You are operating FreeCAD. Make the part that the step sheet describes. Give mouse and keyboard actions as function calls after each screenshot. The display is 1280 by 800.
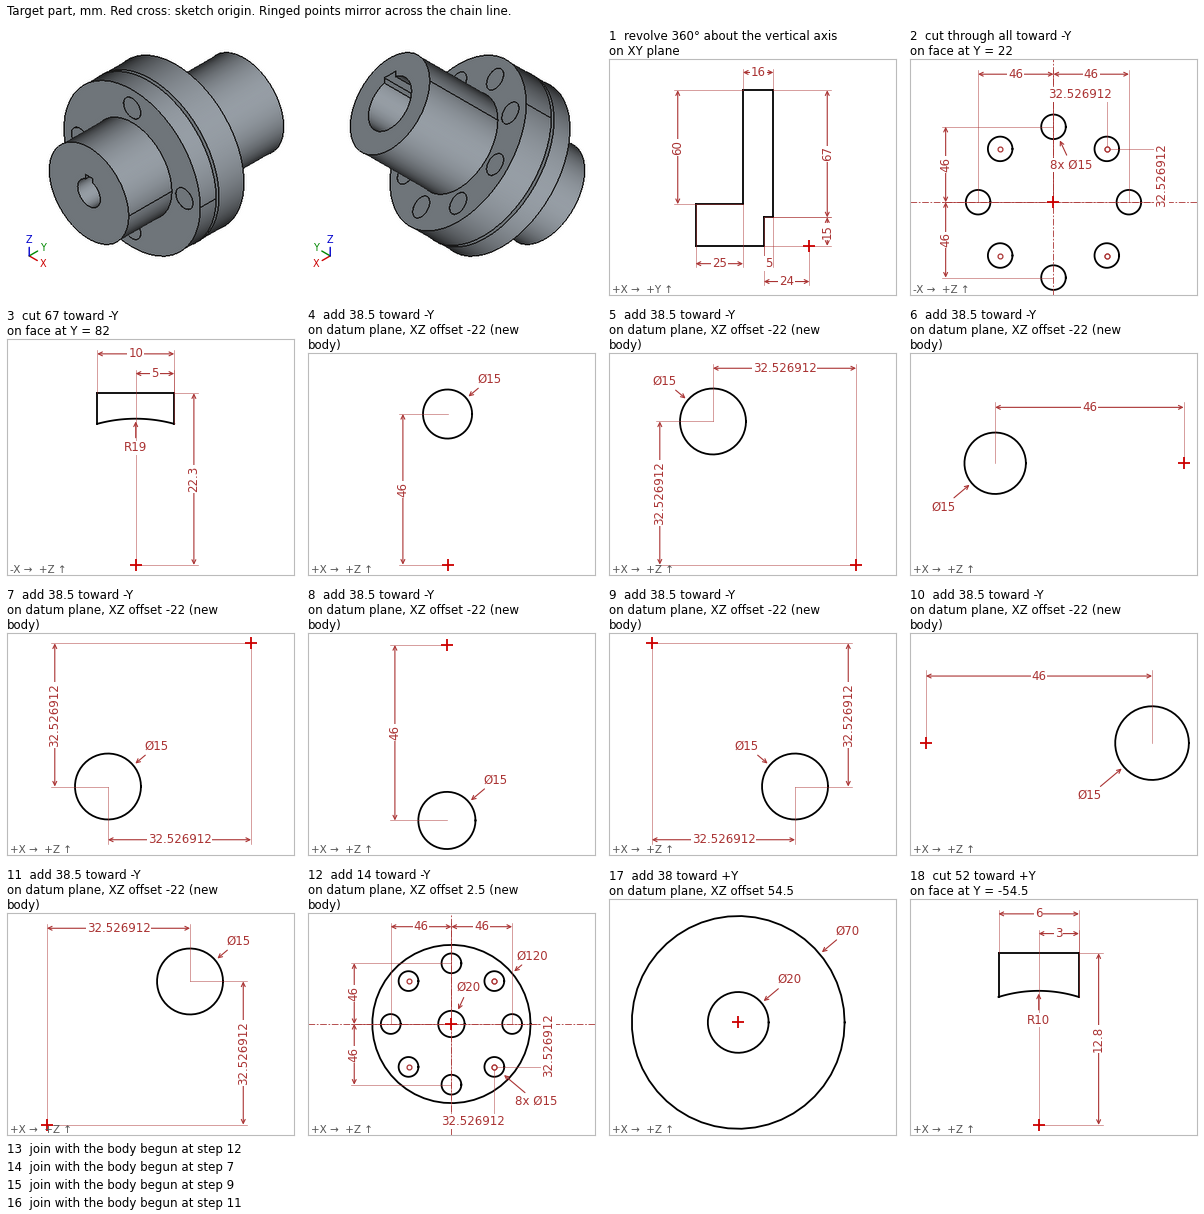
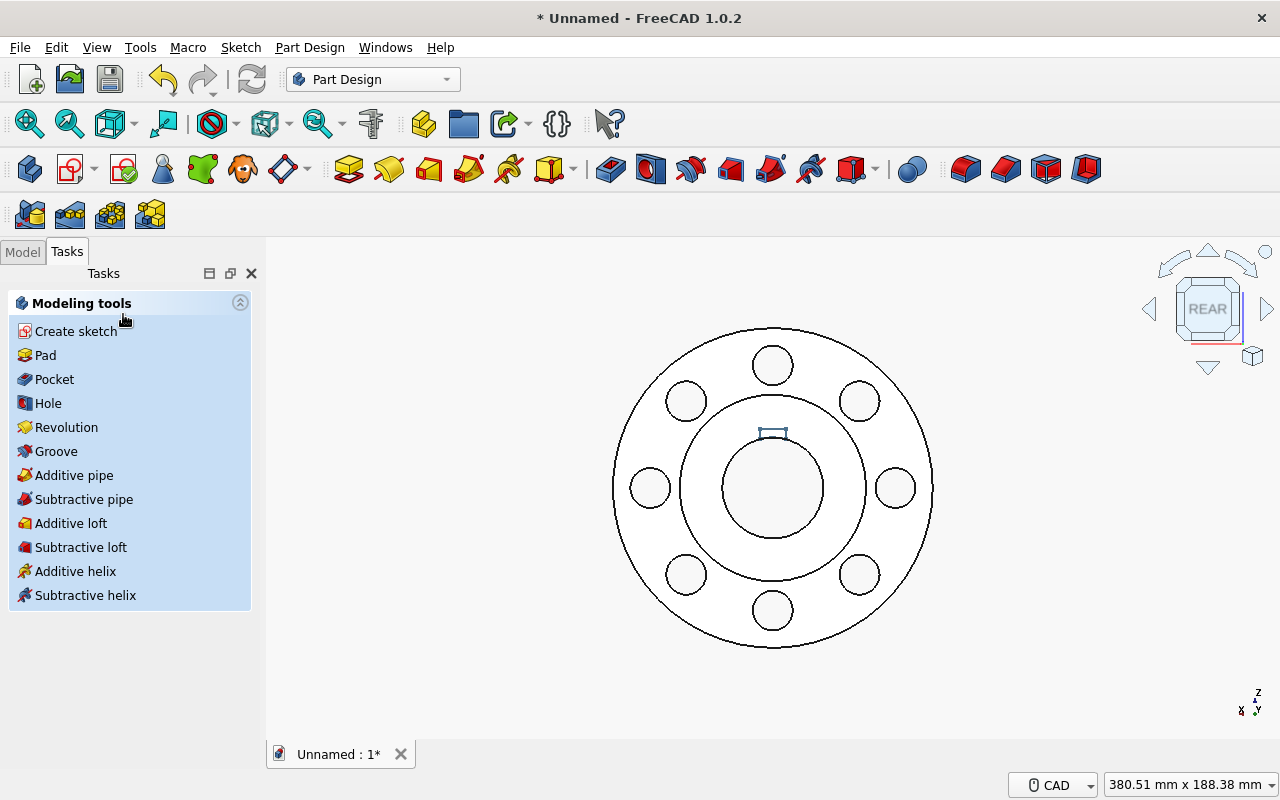
click(612, 170)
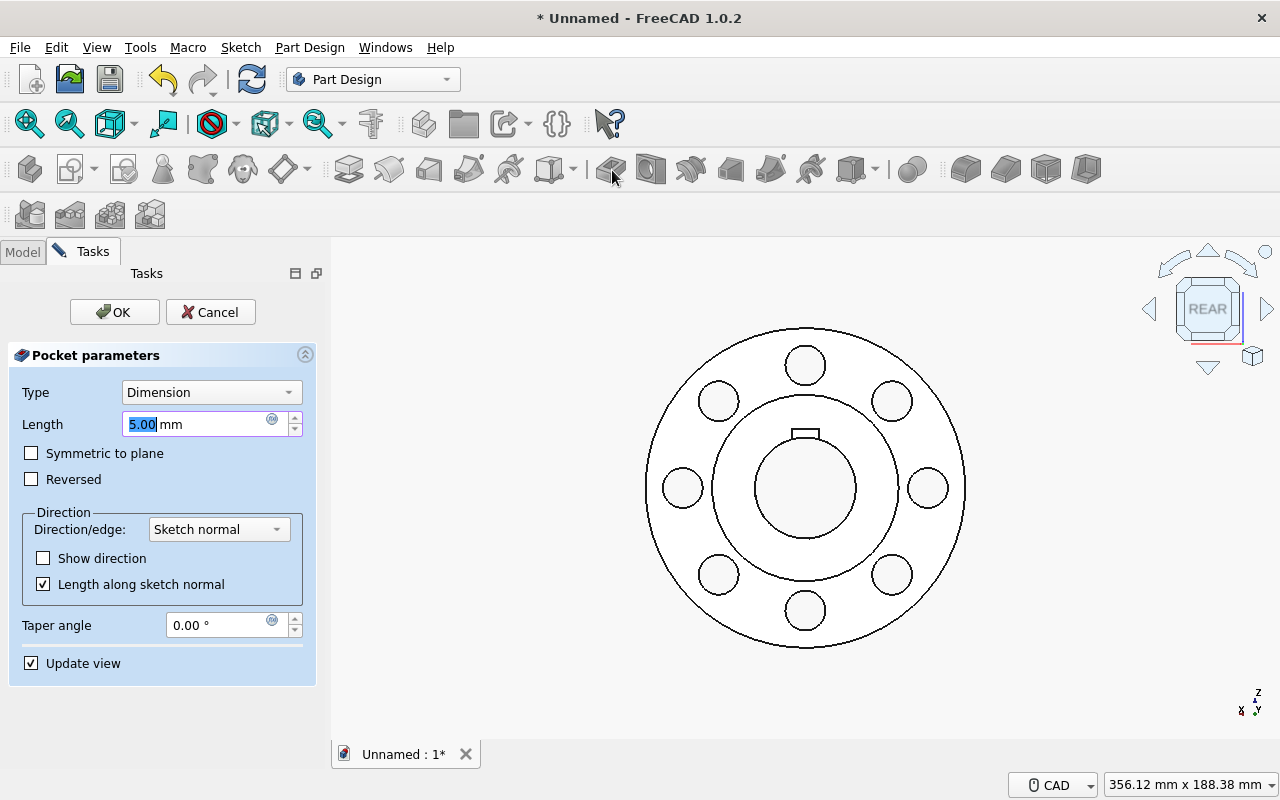
text(67)
key(Tab)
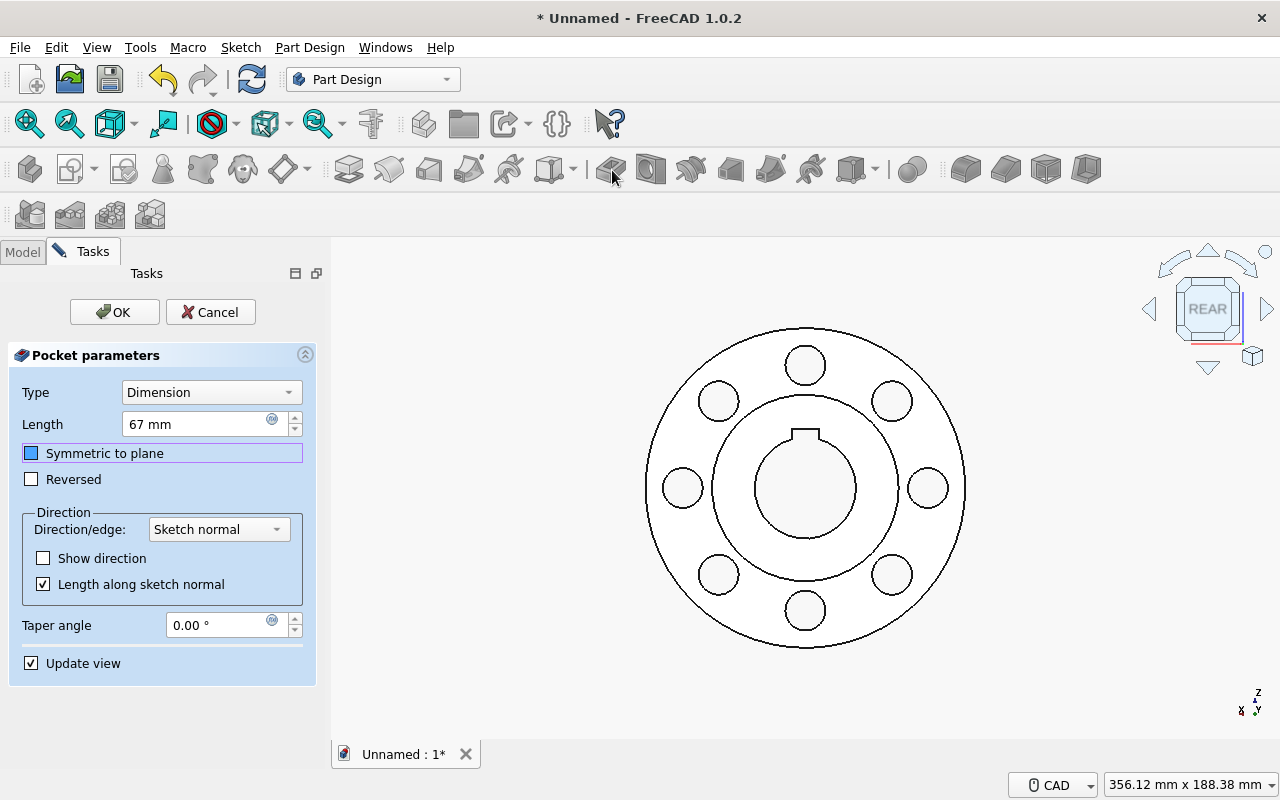
click(115, 312)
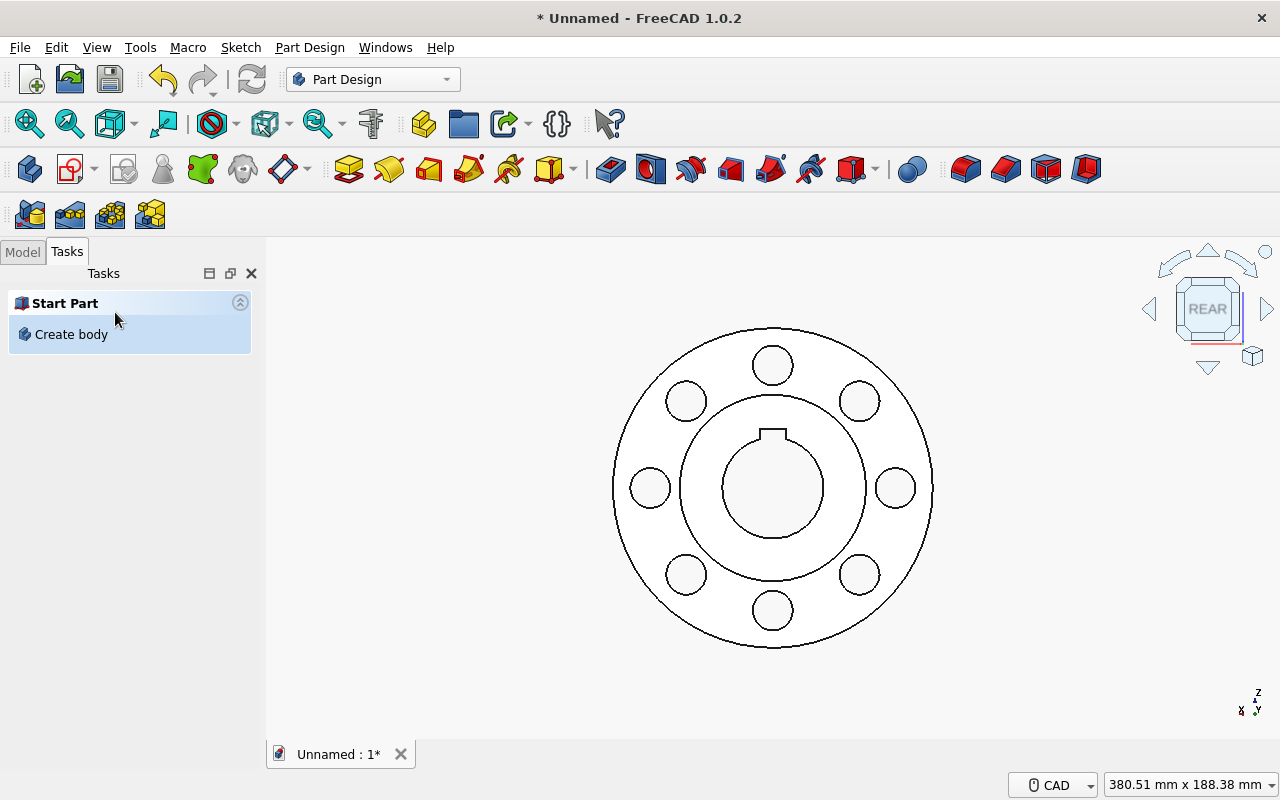
click(30, 170)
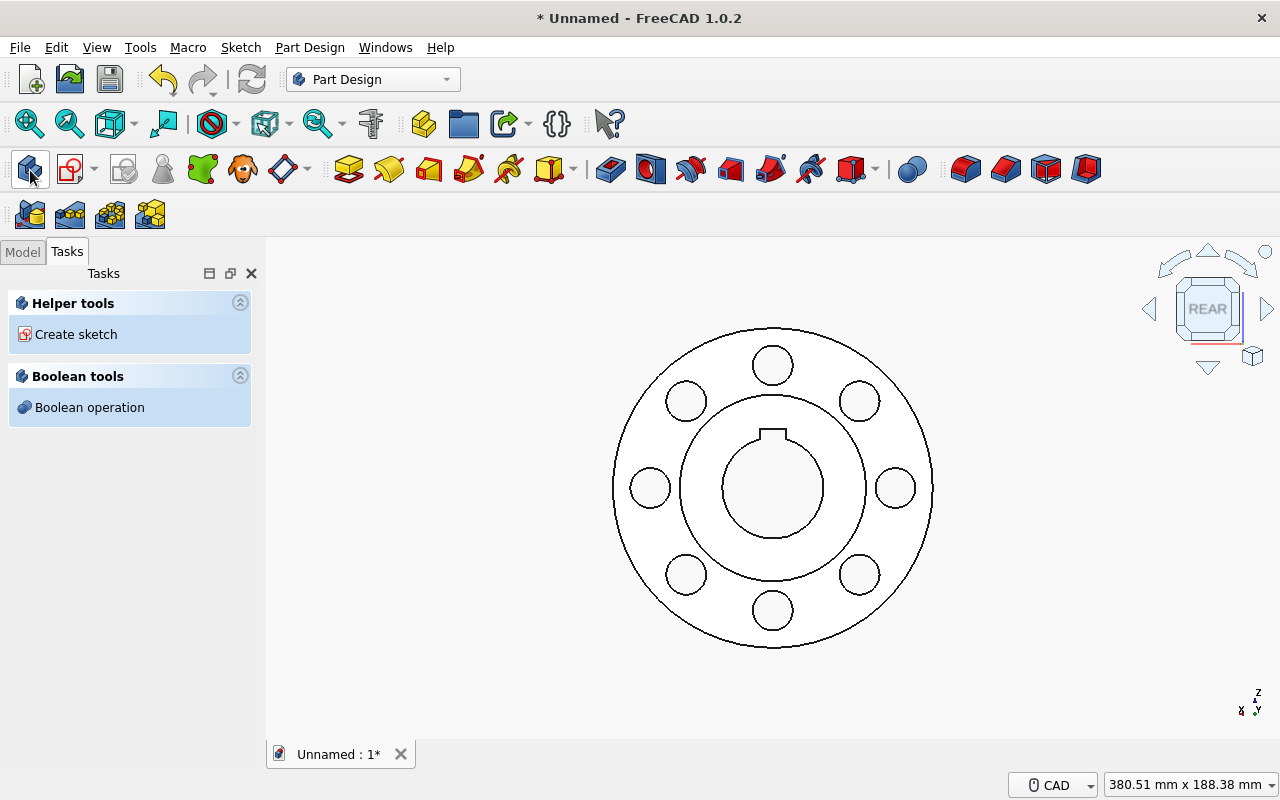
click(23, 251)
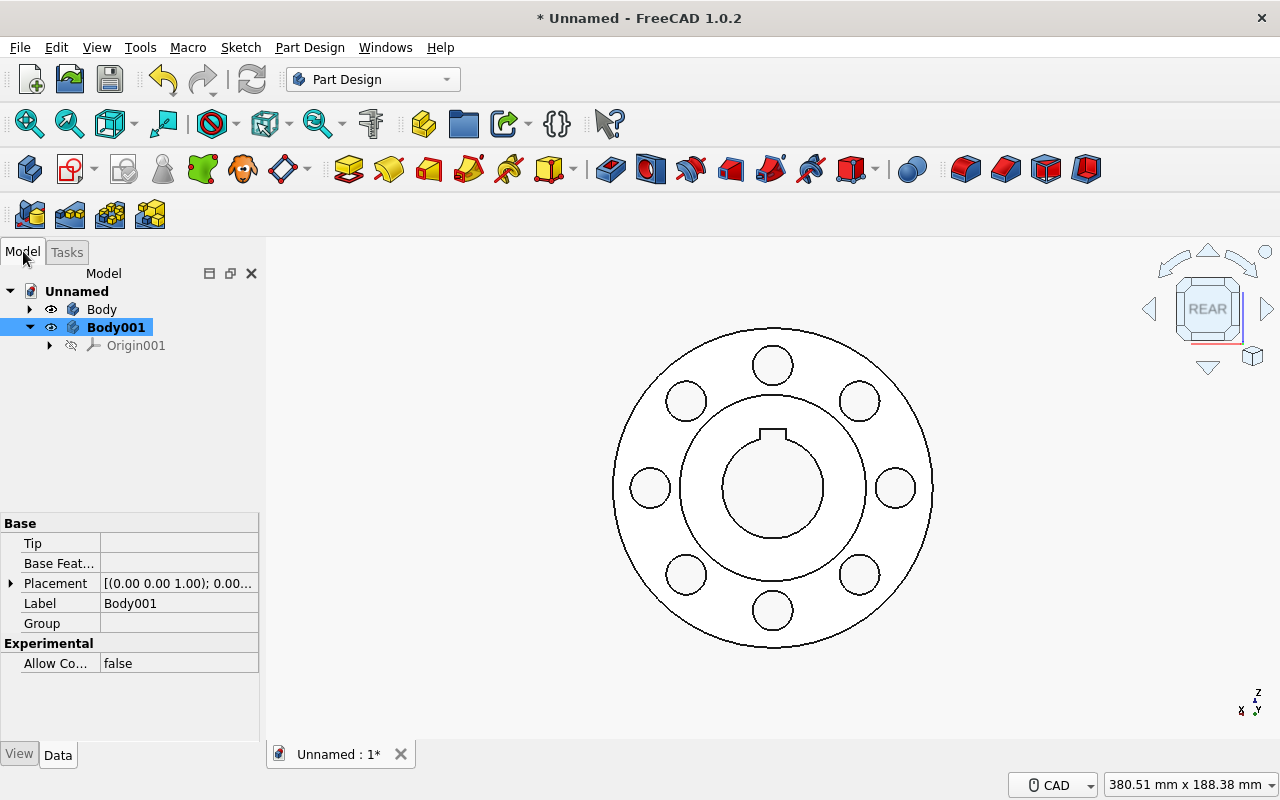
click(50, 345)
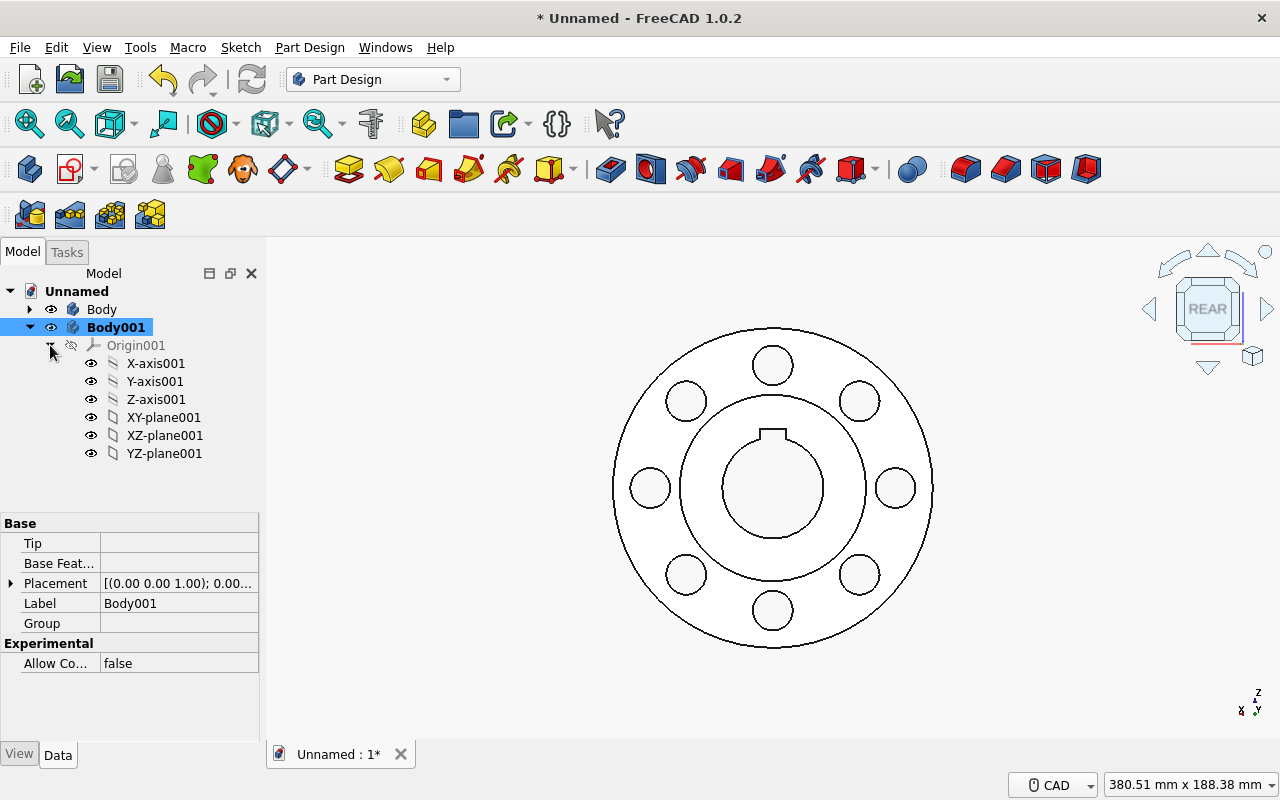
click(136, 435)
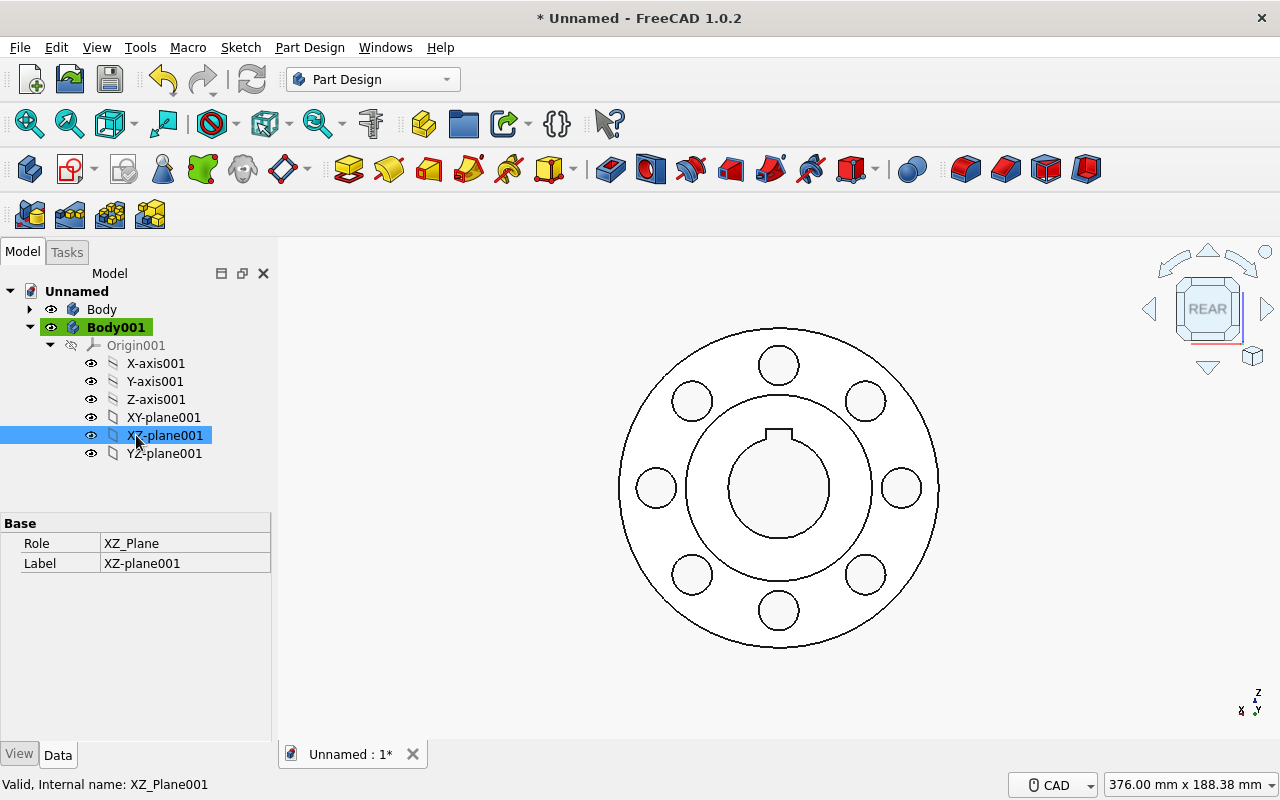
click(284, 170)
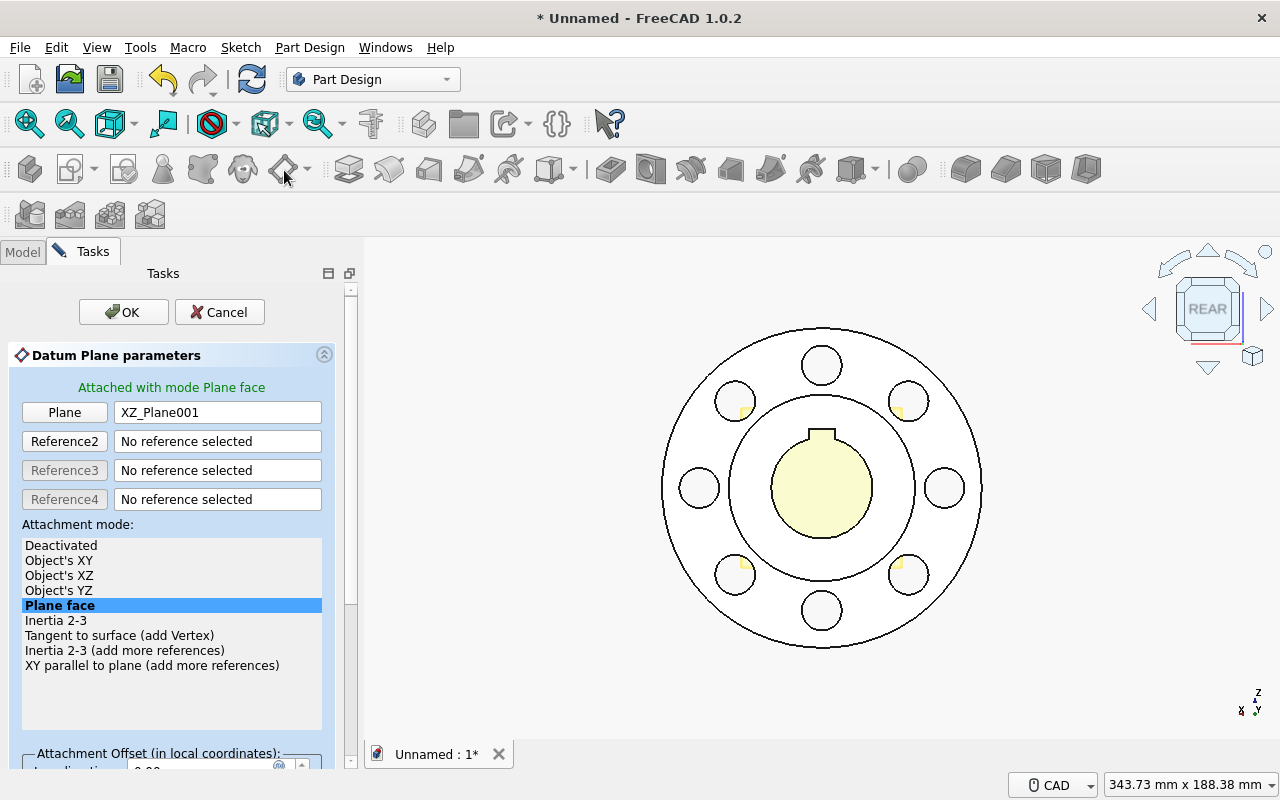
scroll(351, 526, down, 3)